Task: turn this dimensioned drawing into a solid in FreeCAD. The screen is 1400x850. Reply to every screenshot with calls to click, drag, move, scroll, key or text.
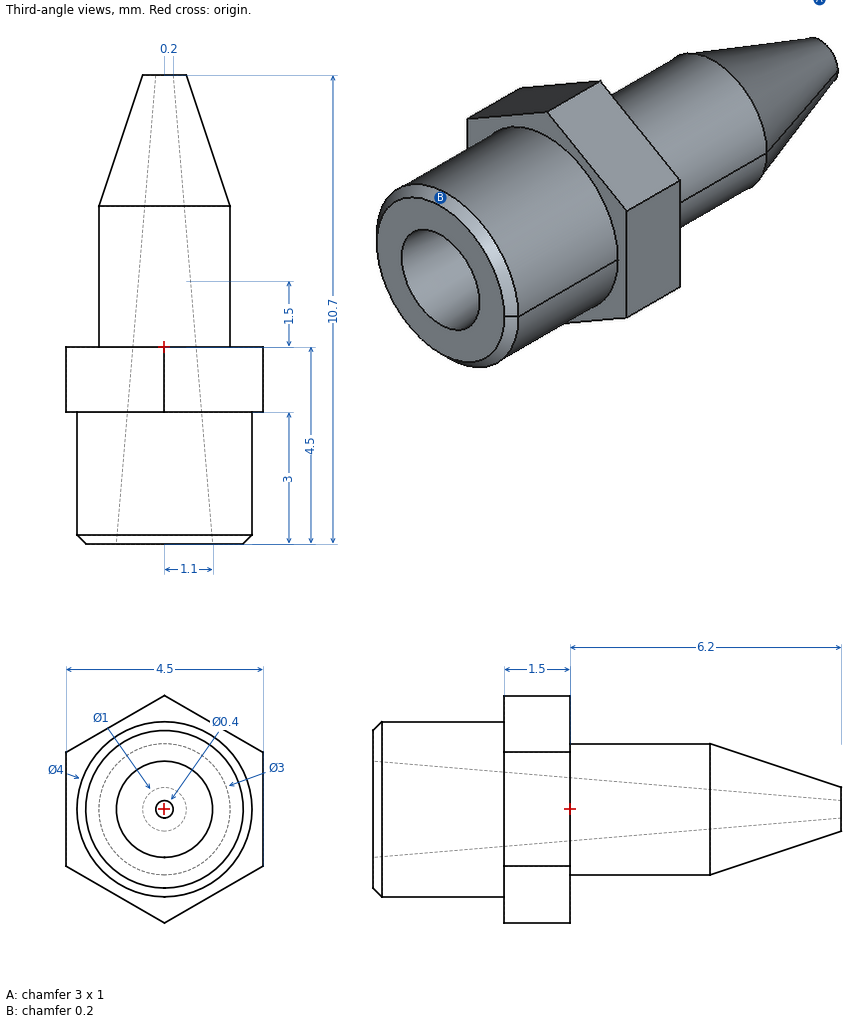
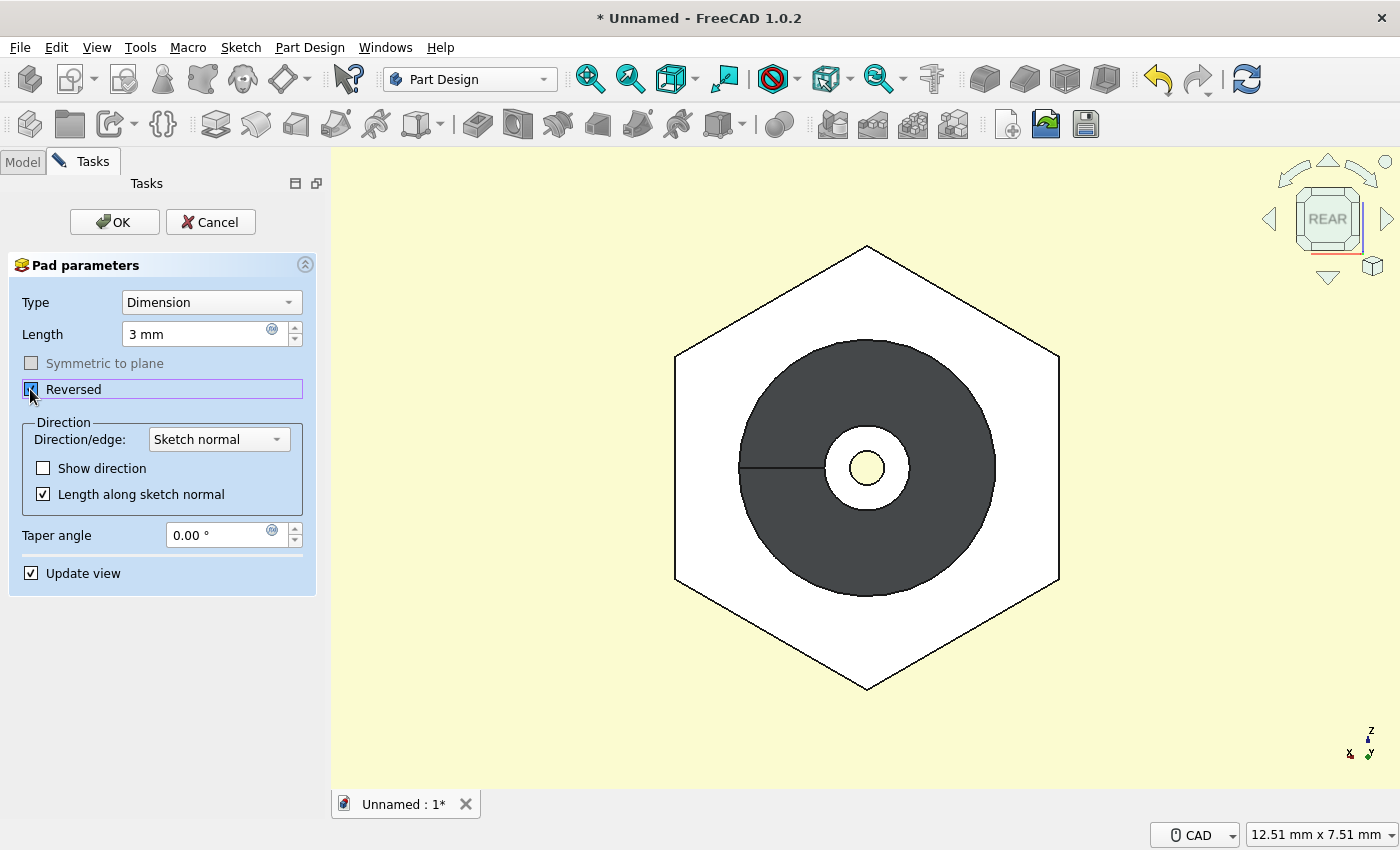
click(115, 222)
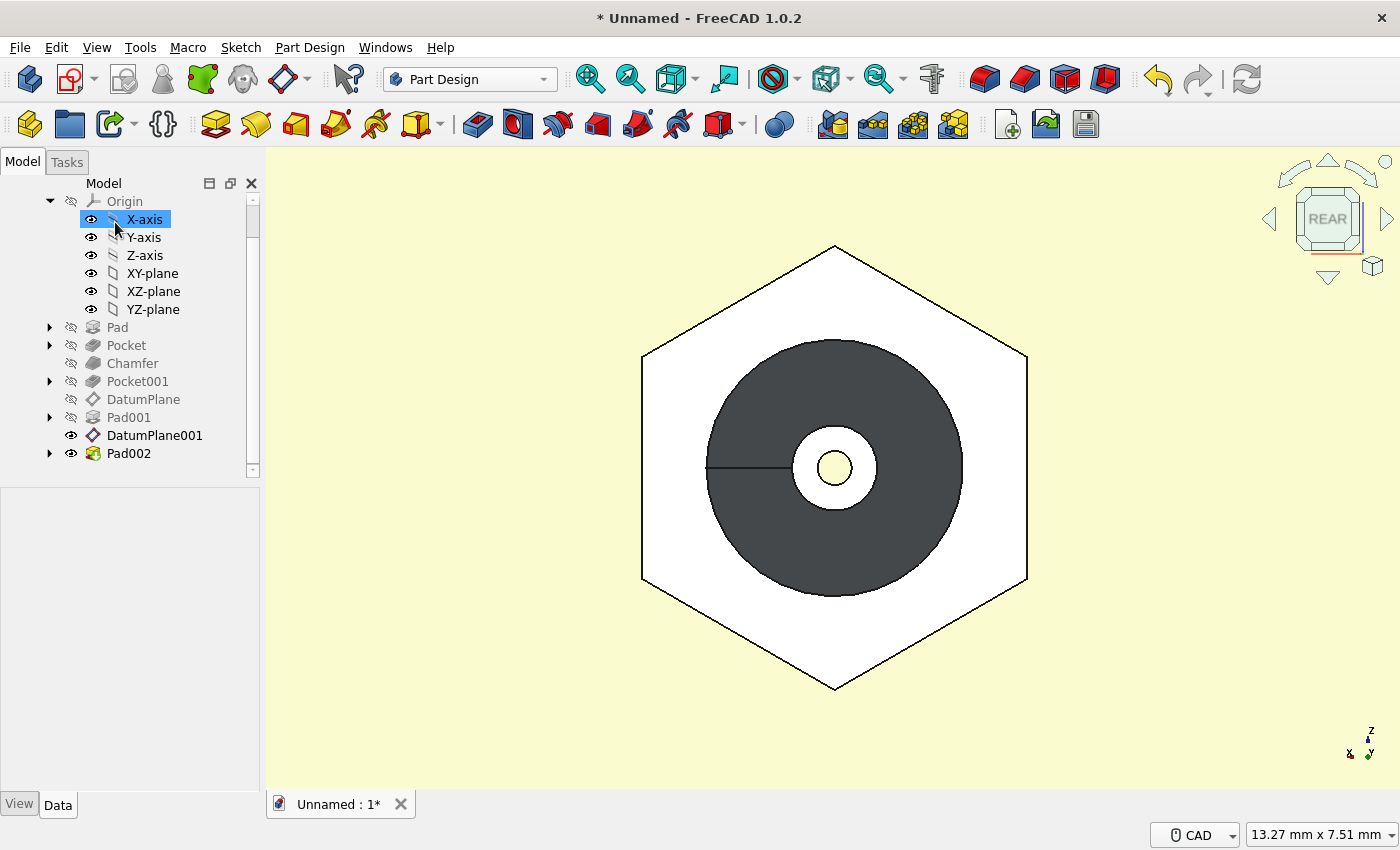
click(116, 435)
key(space)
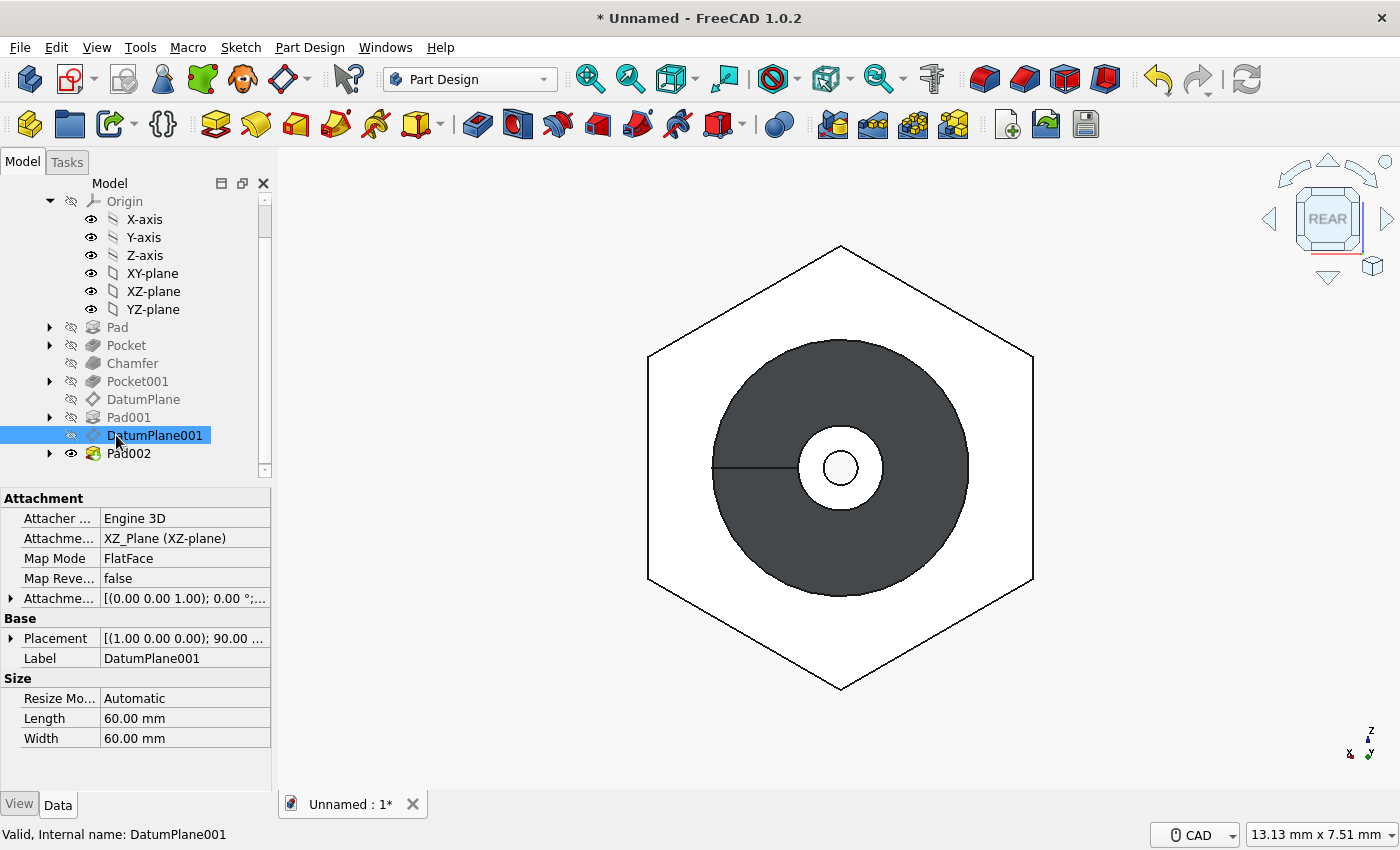
click(318, 749)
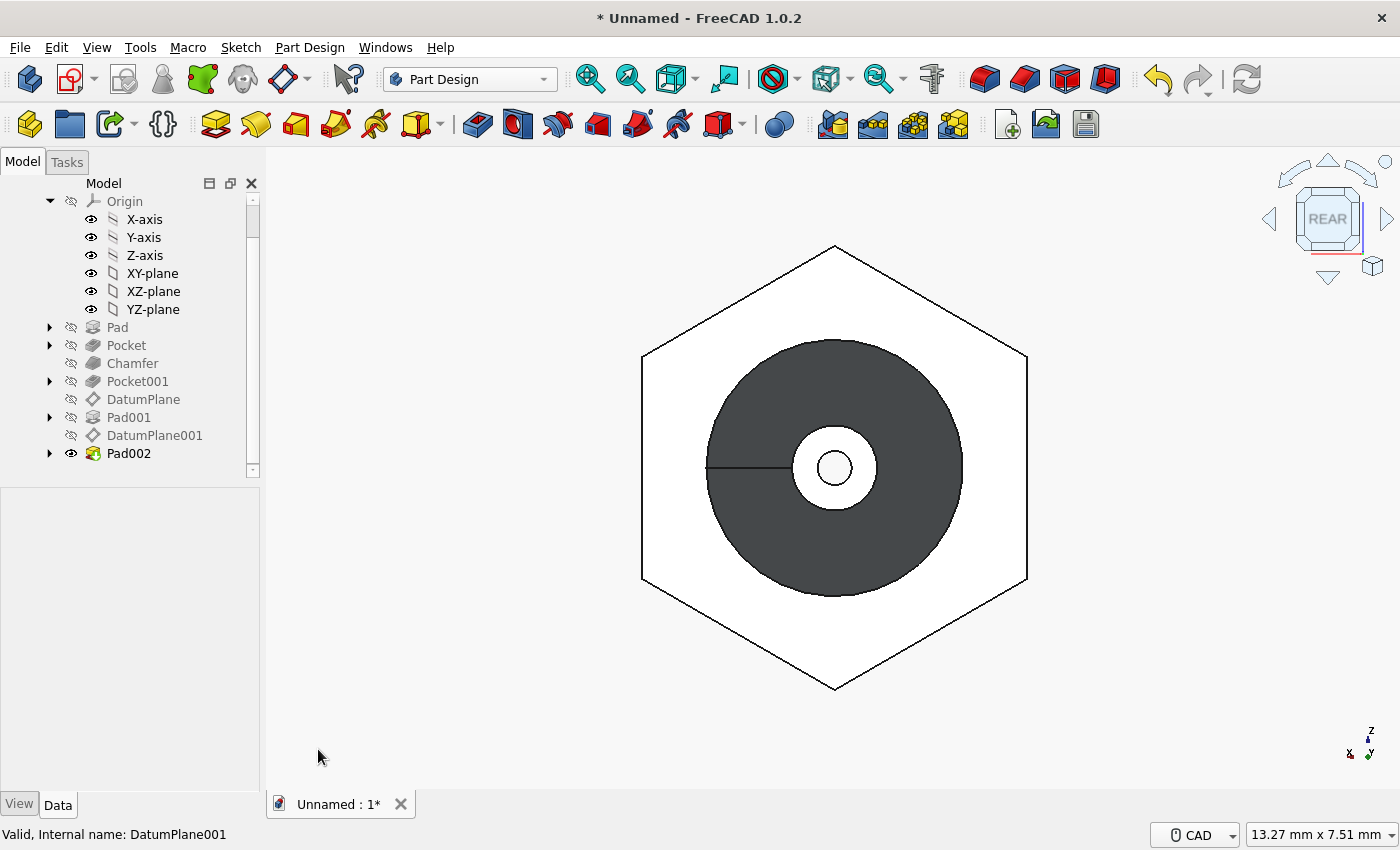
click(70, 80)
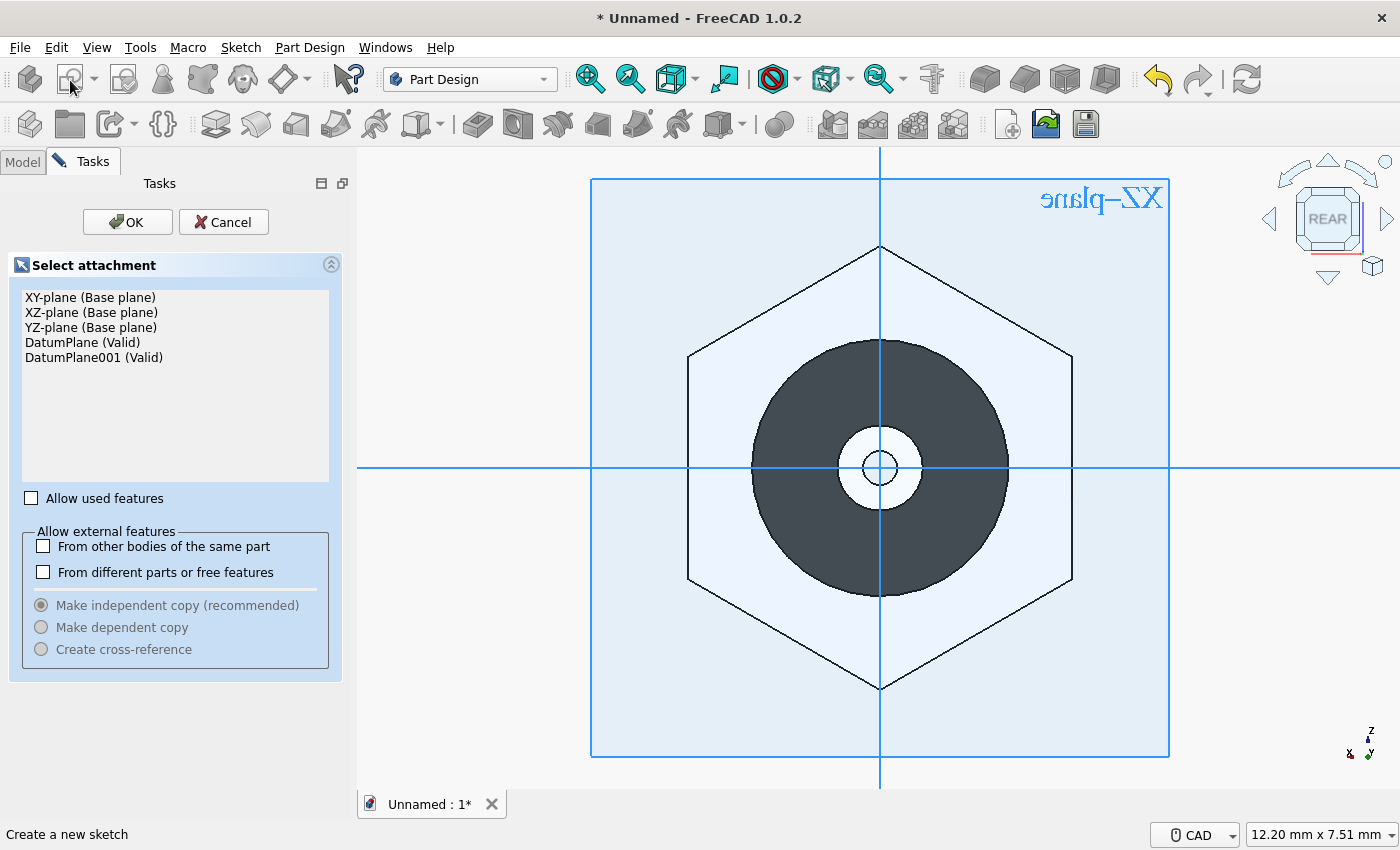
click(82, 298)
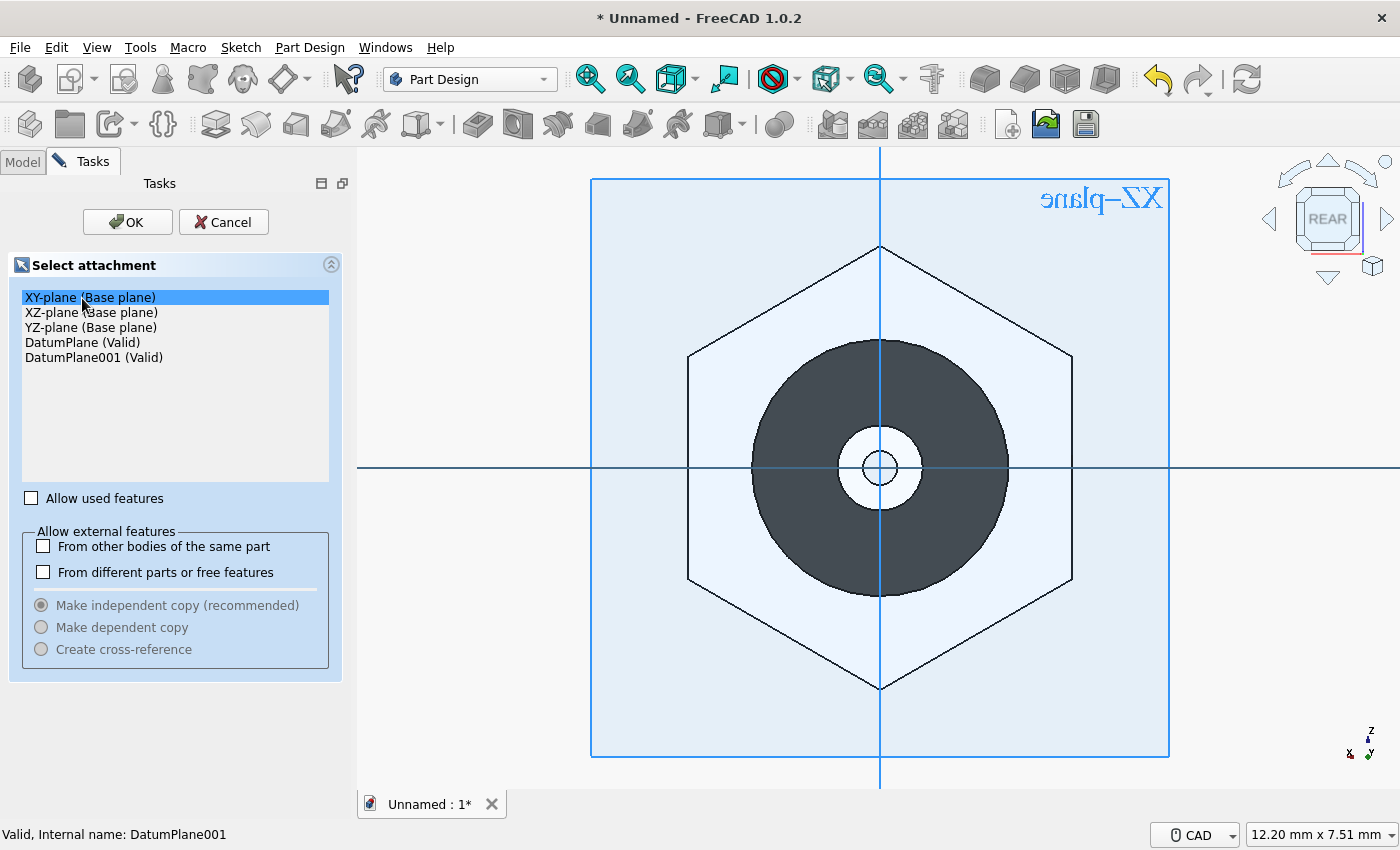
click(128, 222)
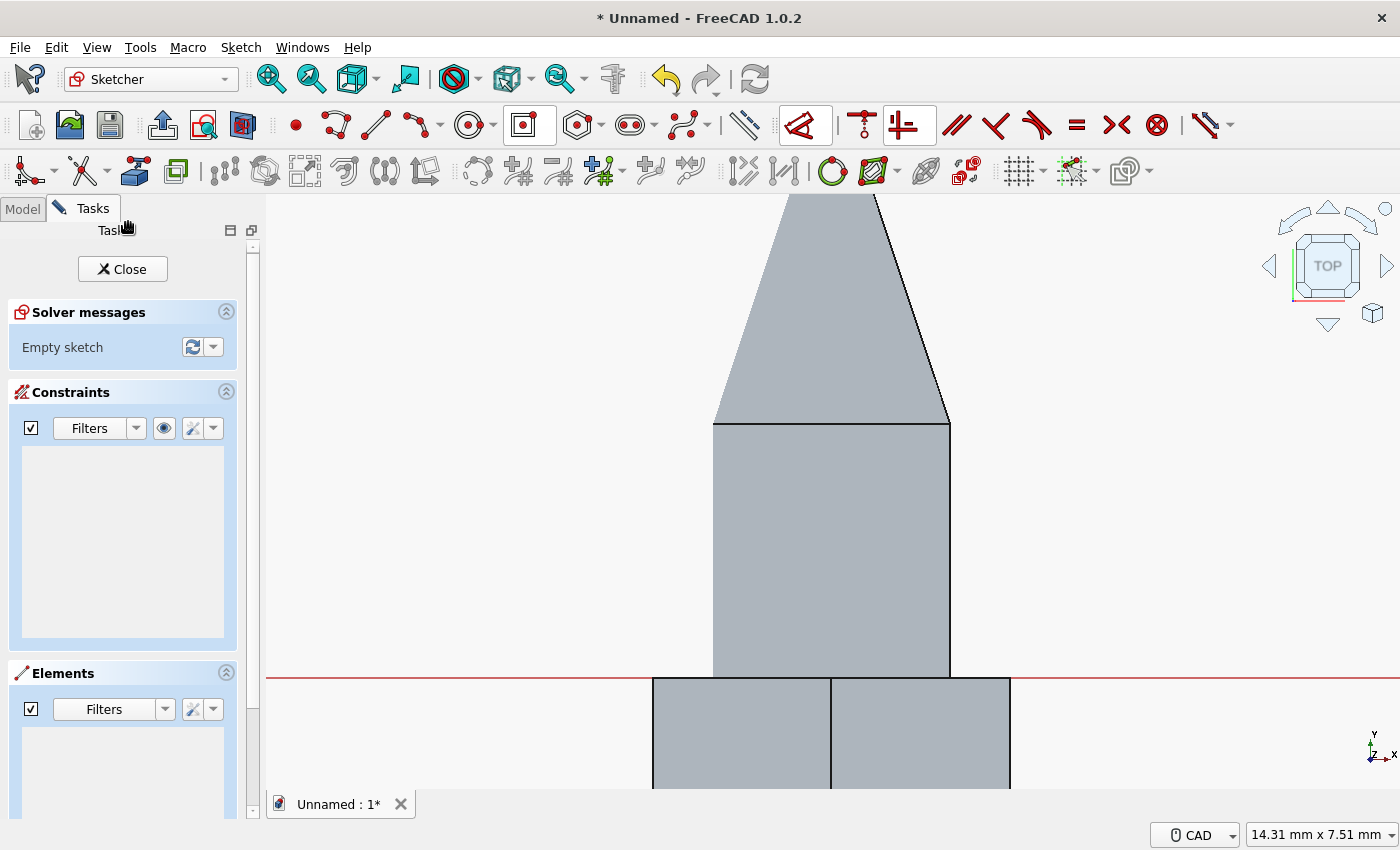
click(244, 126)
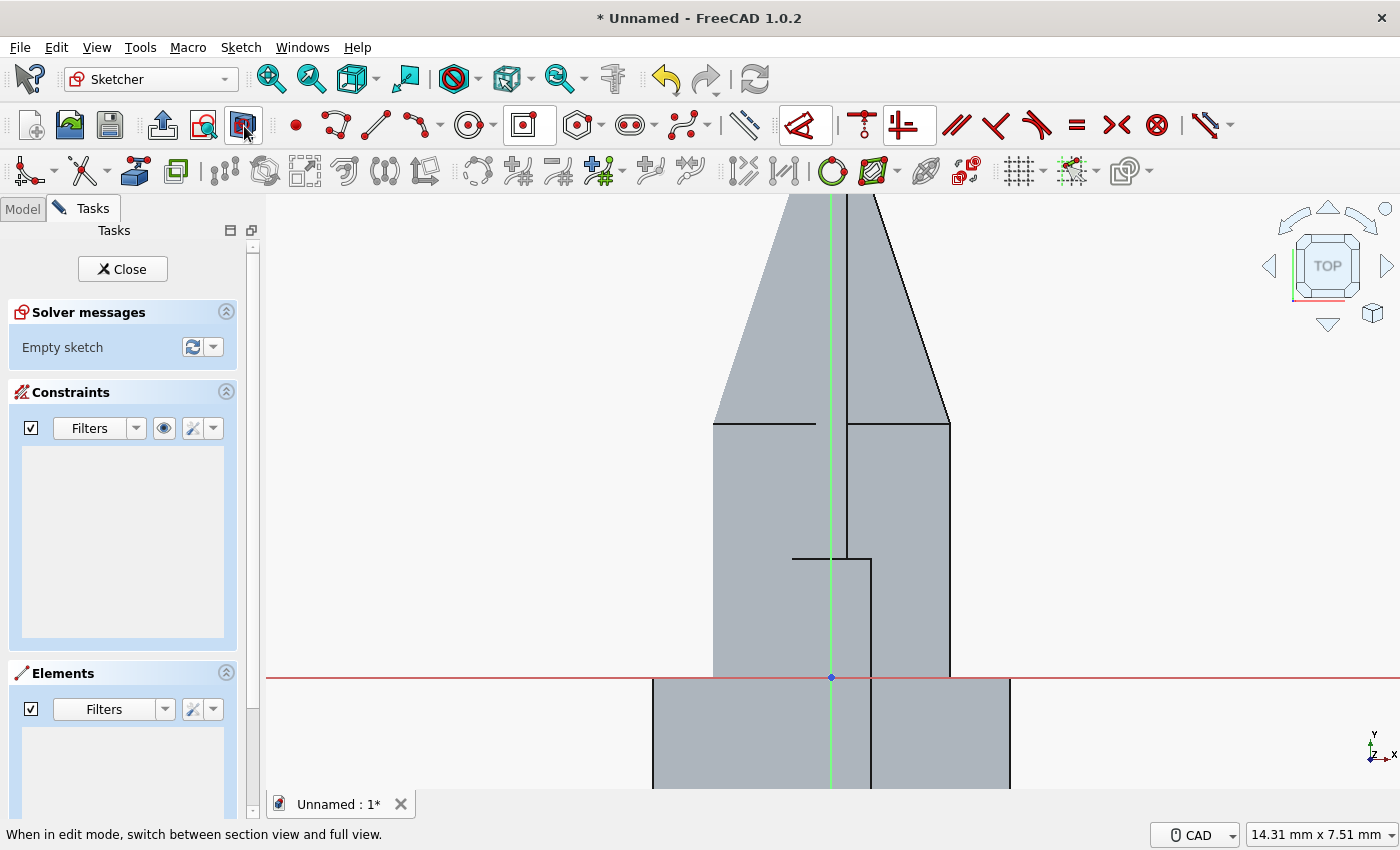
scroll(674, 395, down, 4)